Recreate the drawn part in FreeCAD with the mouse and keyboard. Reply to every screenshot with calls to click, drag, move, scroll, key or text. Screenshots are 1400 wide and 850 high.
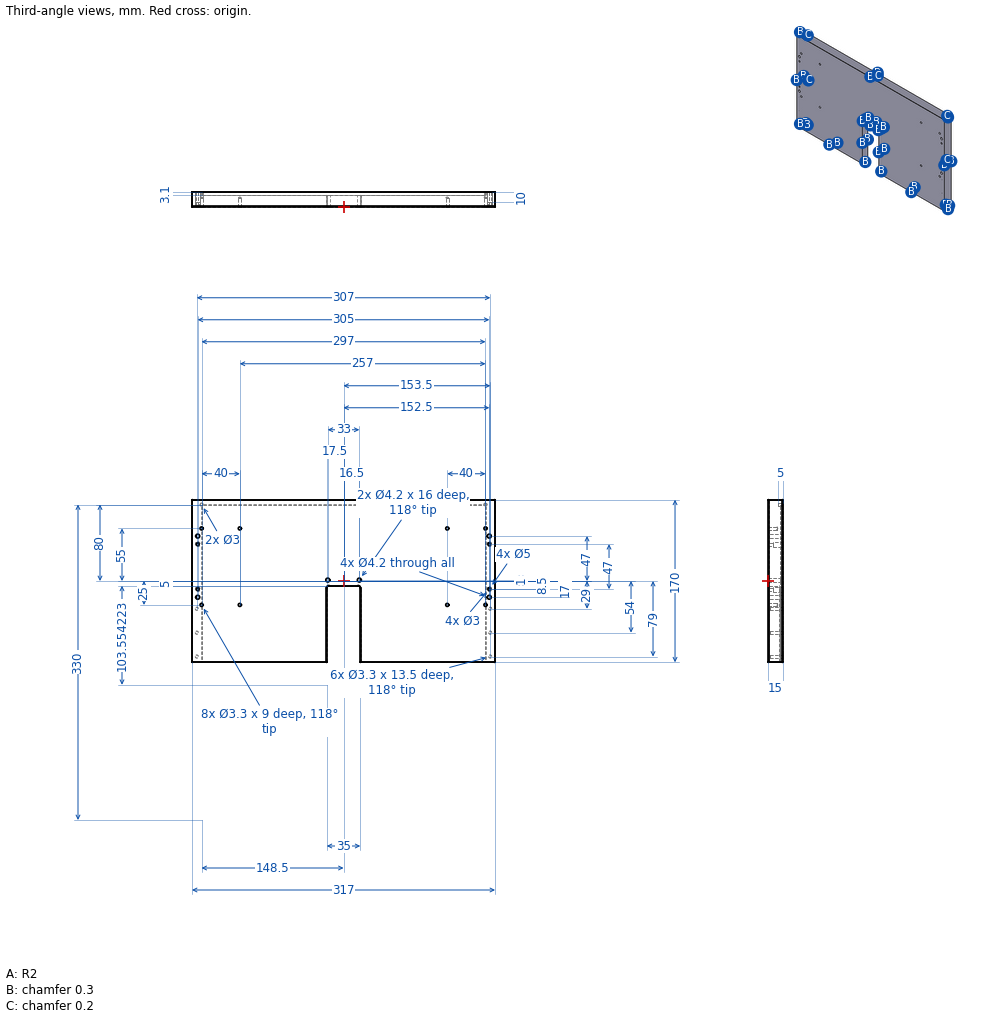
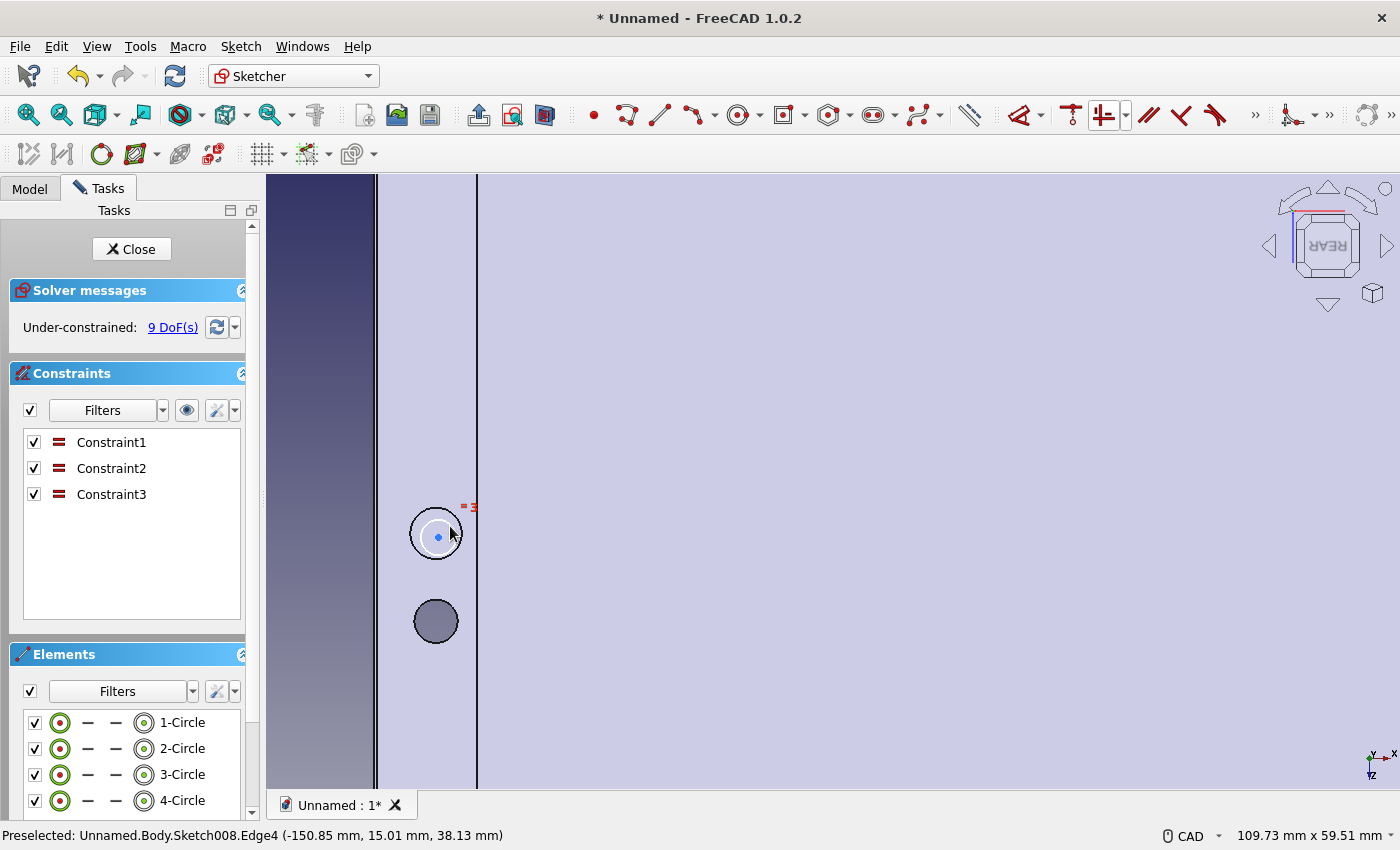
scroll(449, 530, down, 8)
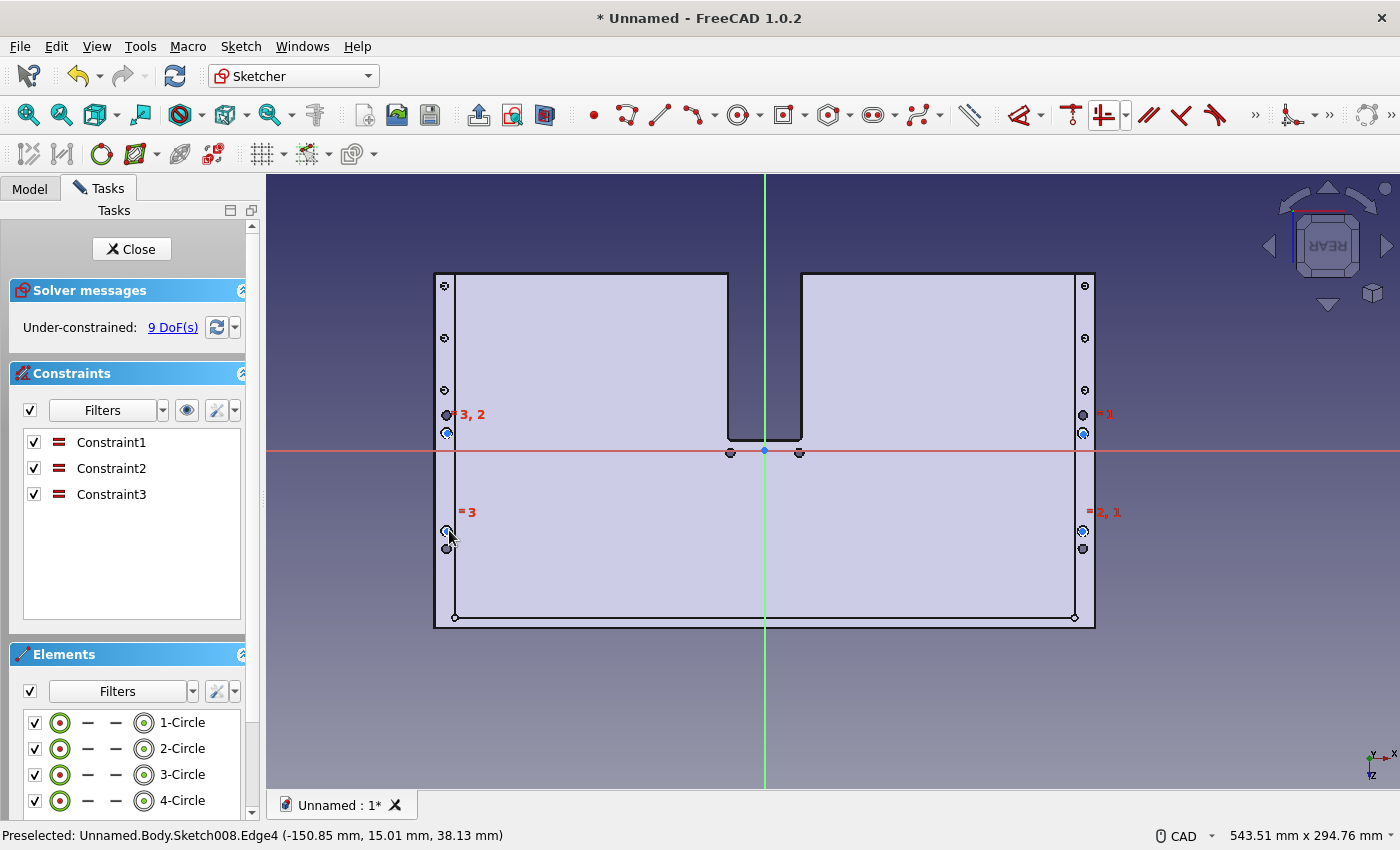
click(1083, 434)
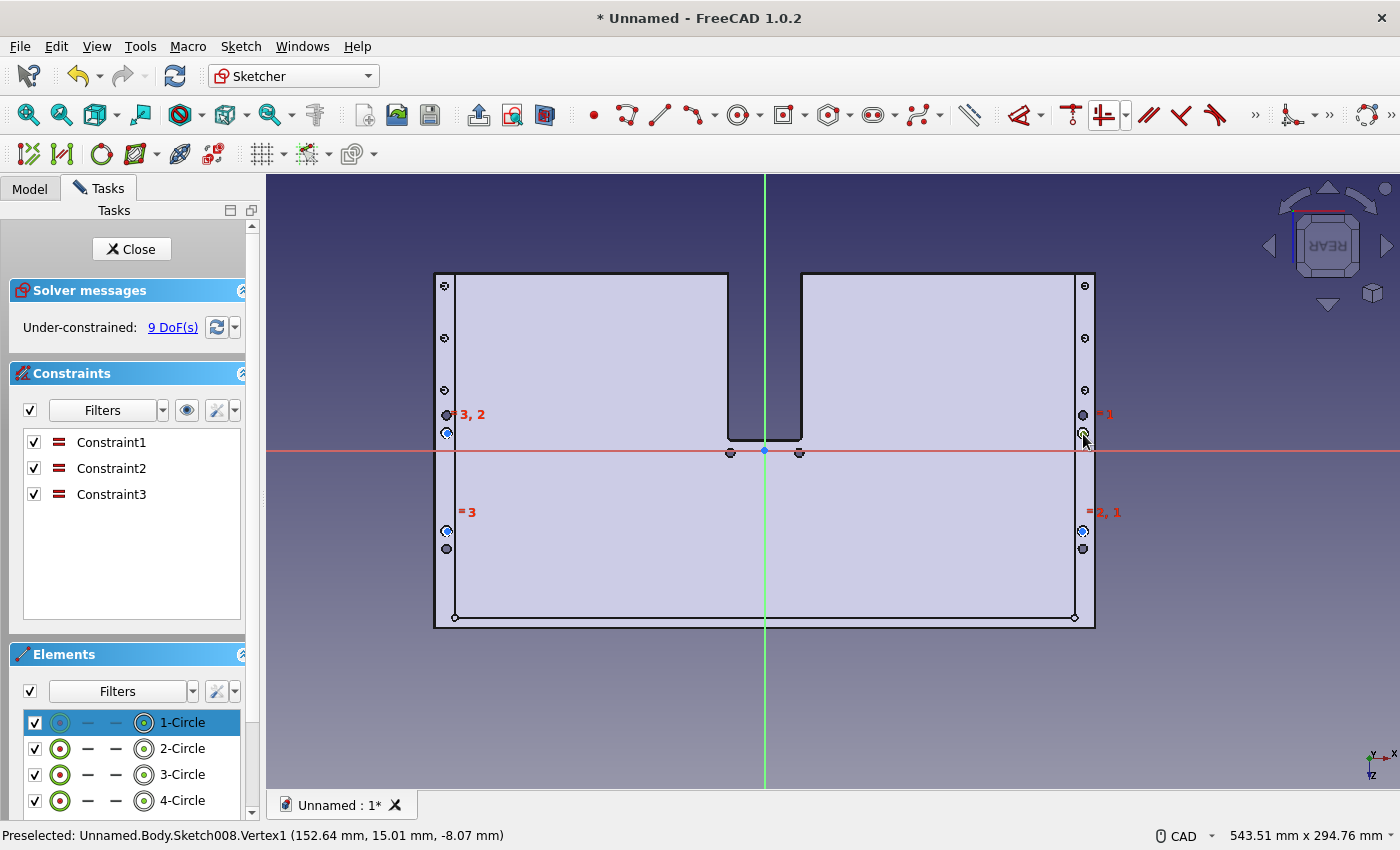
click(1083, 532)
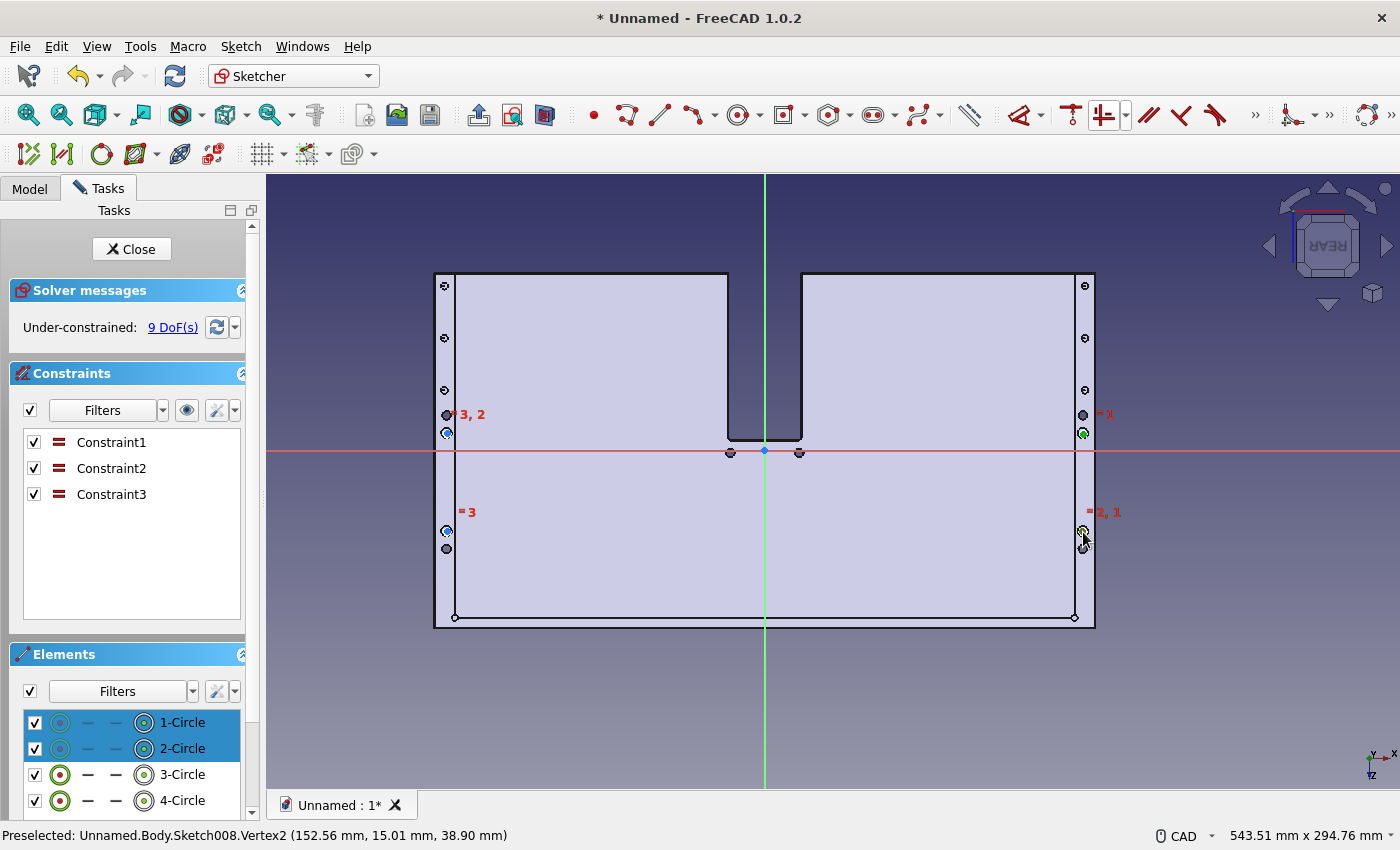
key(v)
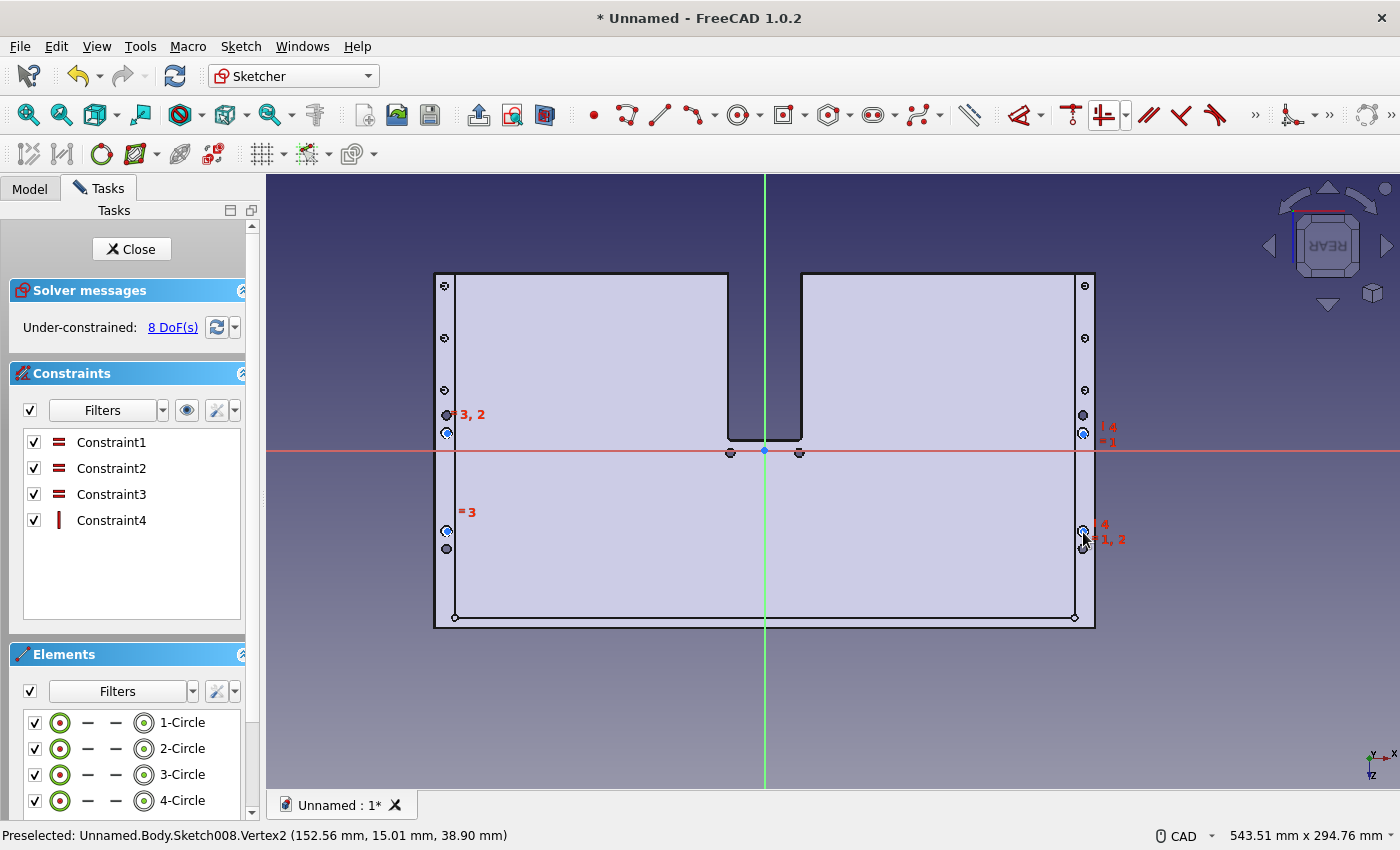
click(1083, 434)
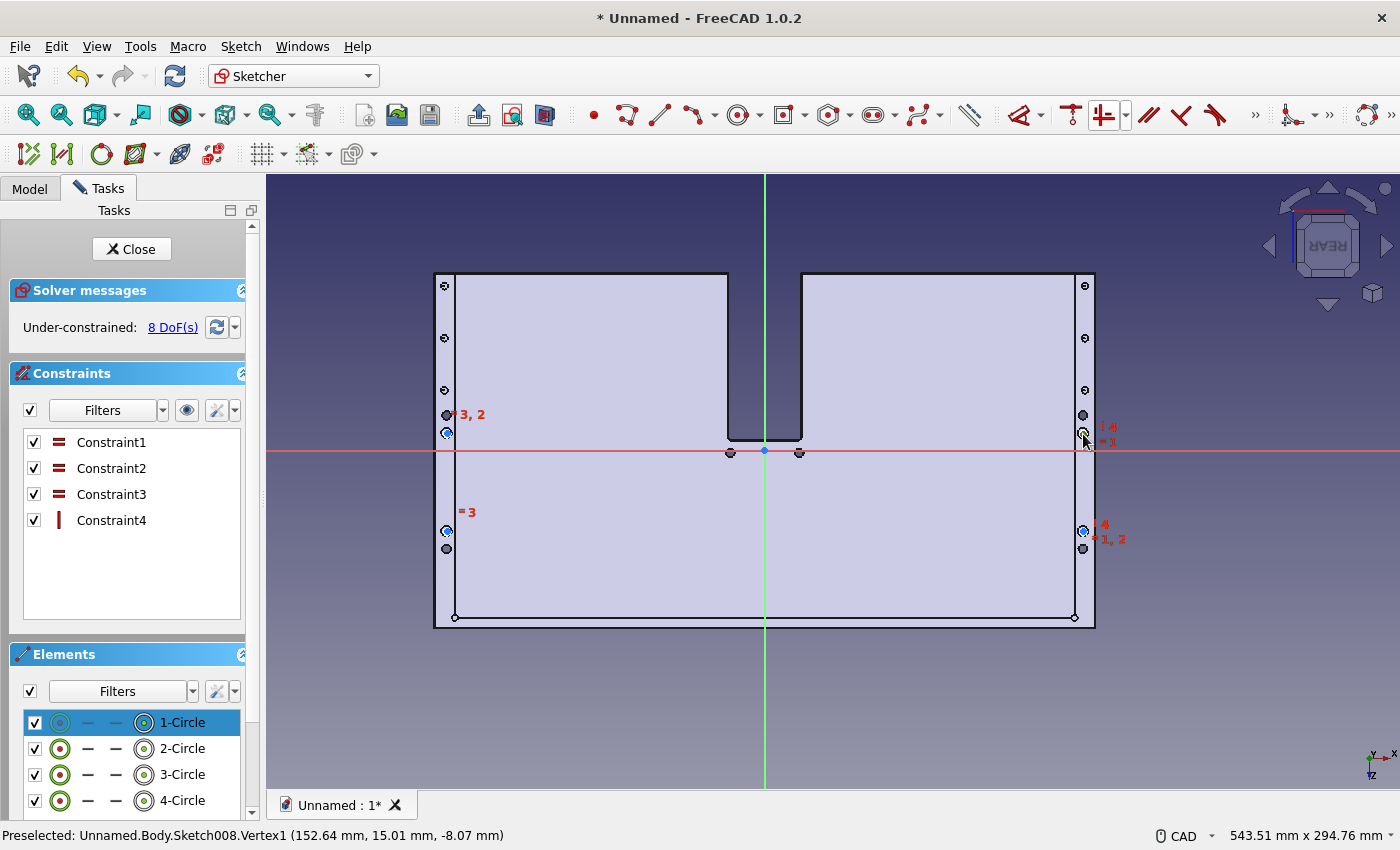
click(447, 434)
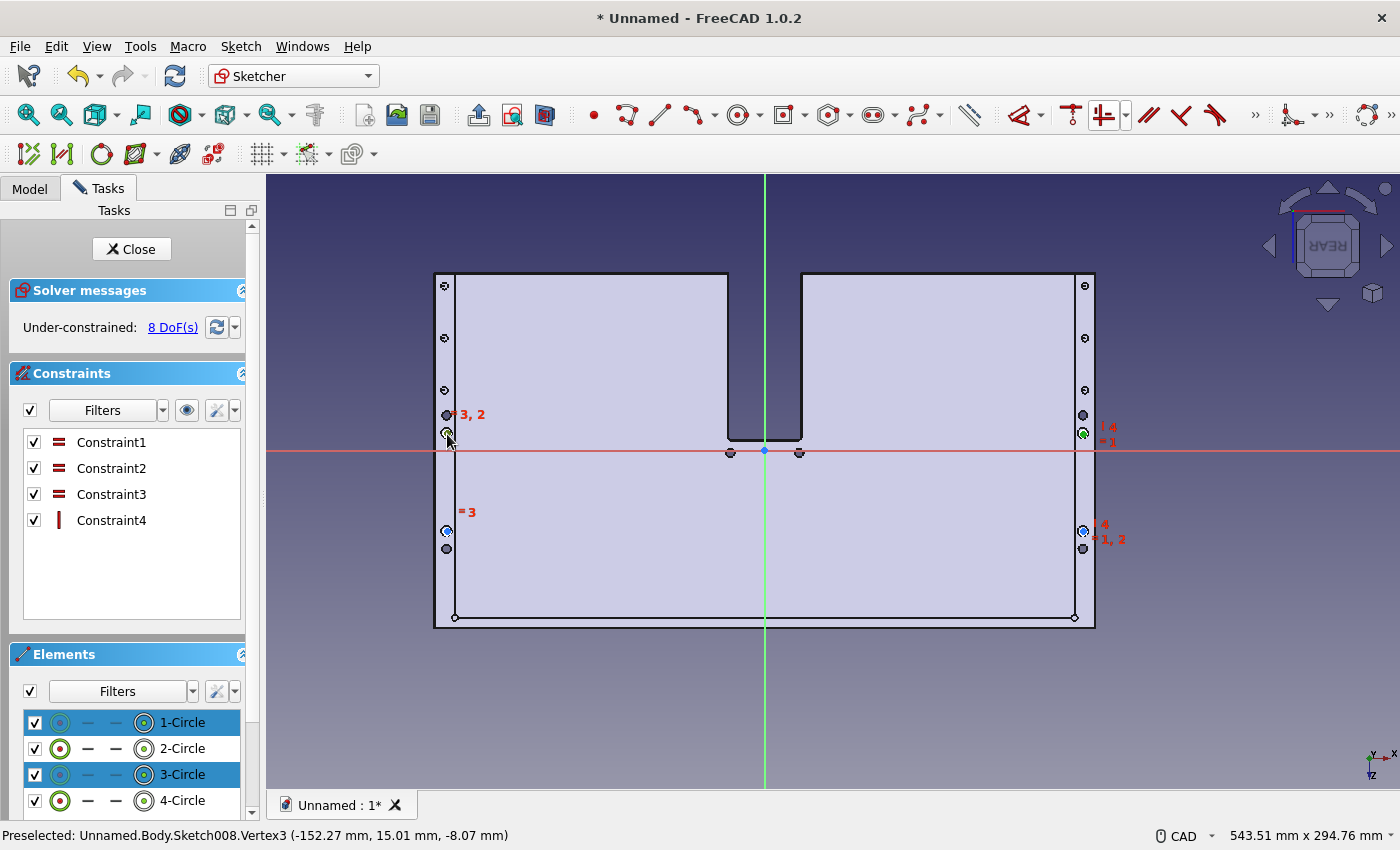
key(h)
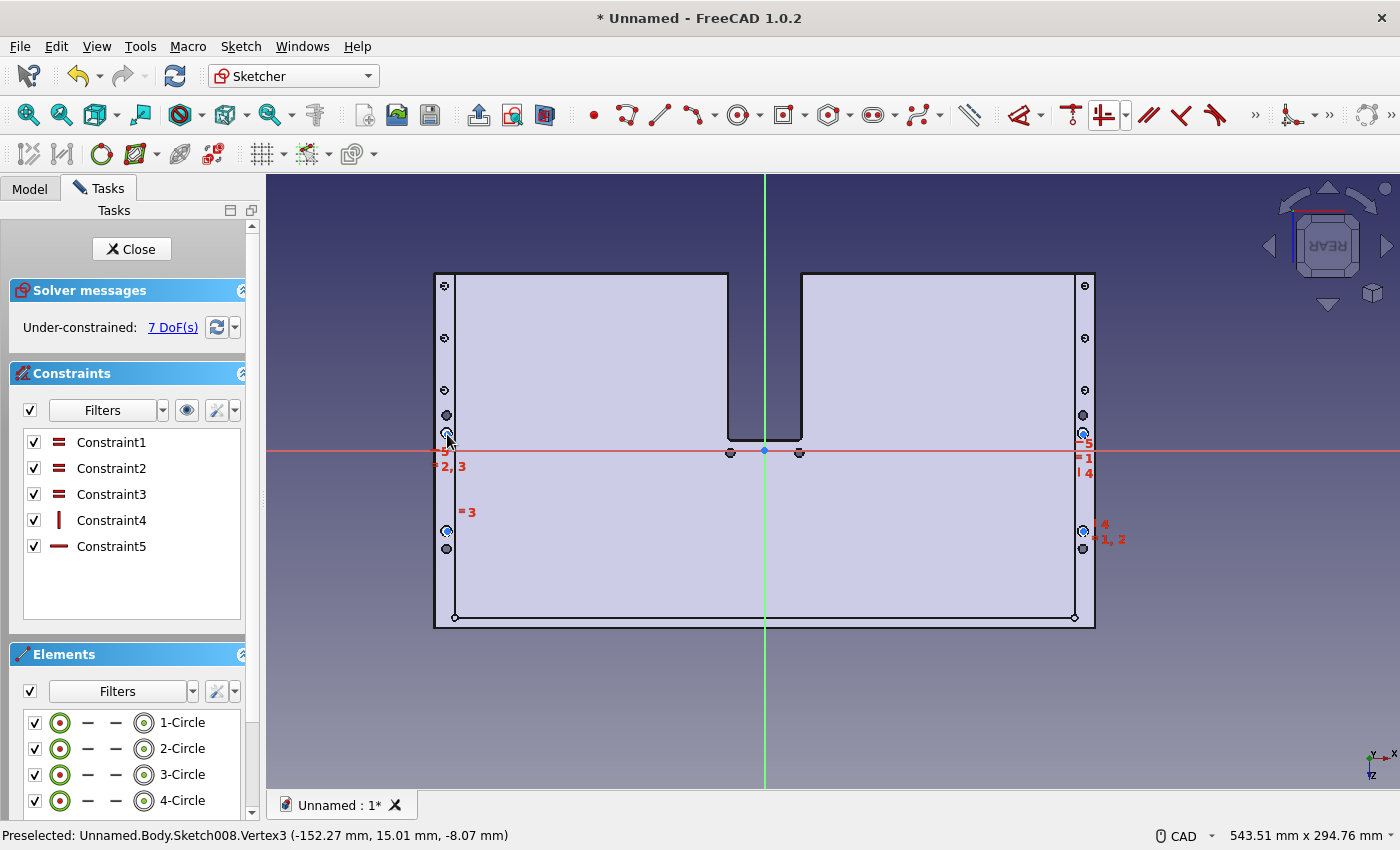
click(447, 434)